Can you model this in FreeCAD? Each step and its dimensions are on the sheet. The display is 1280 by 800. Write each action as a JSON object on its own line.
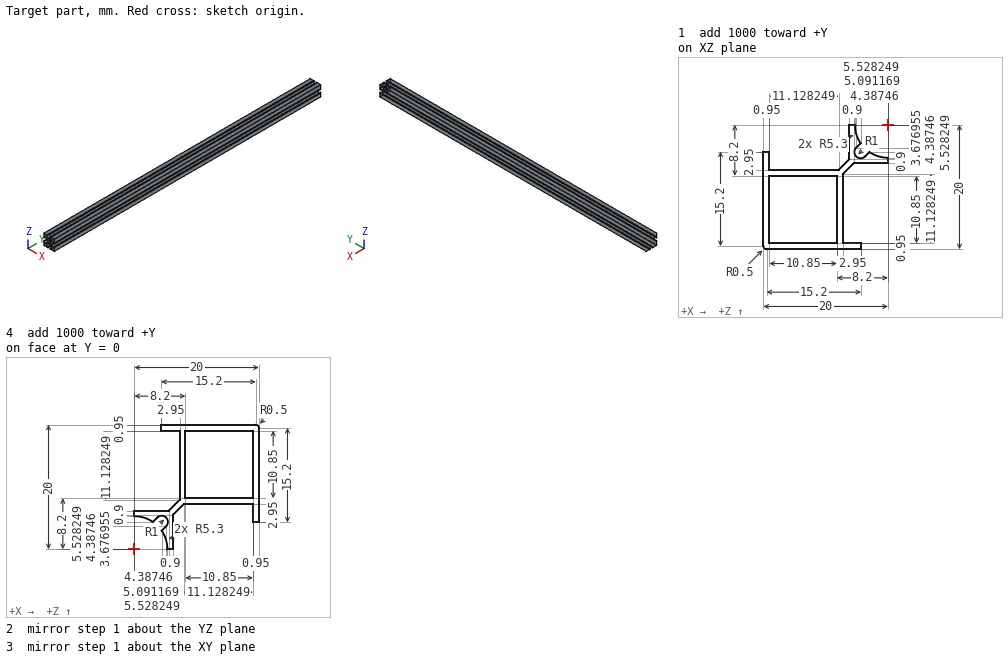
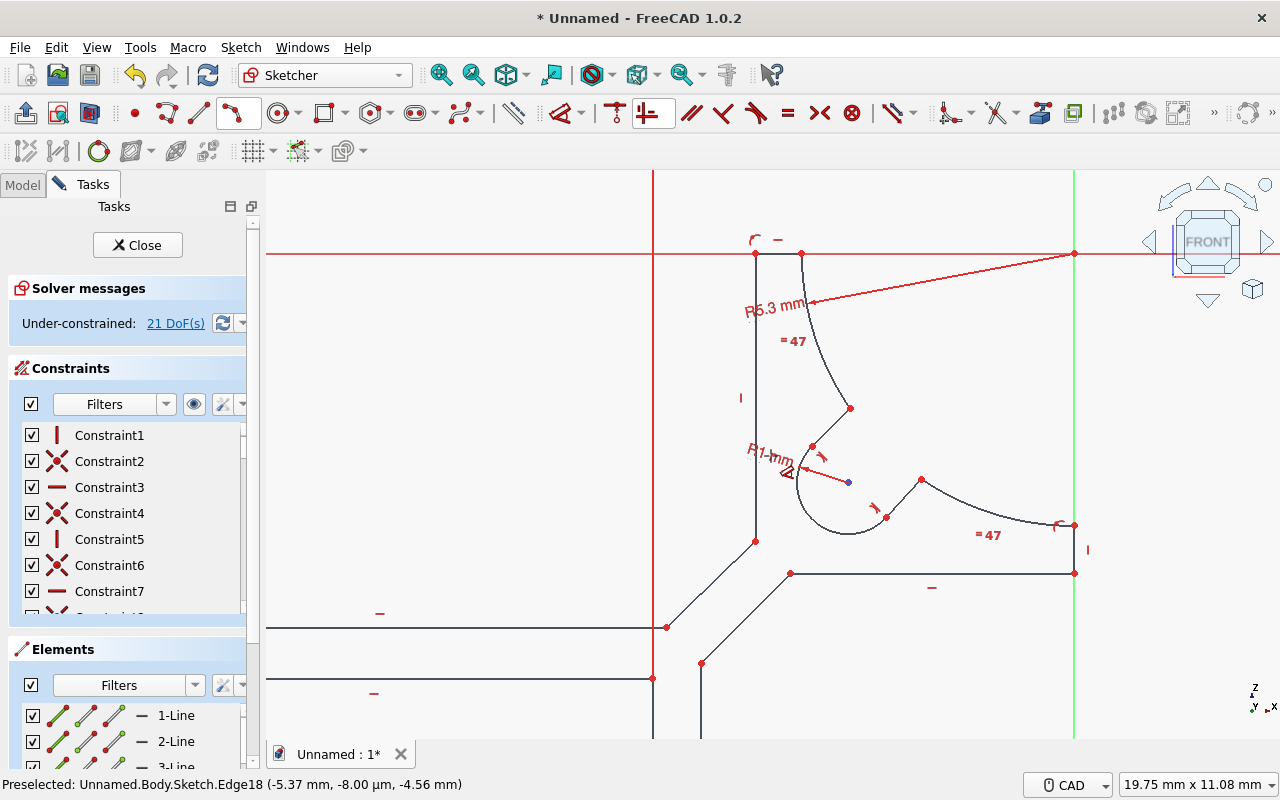
{"action": "scroll", "coordinate": [788, 272], "scroll_direction": "down", "scroll_amount": 5}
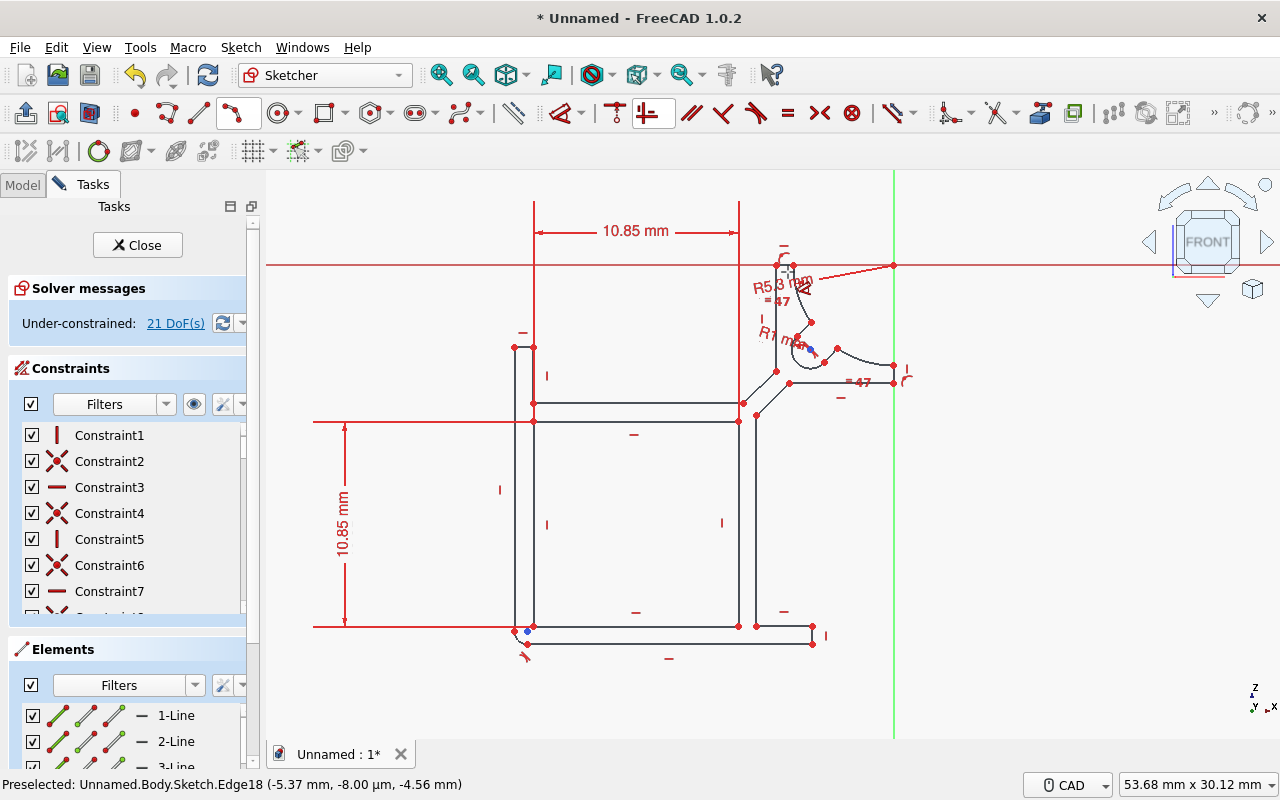
{"action": "scroll", "coordinate": [516, 637], "scroll_direction": "up", "scroll_amount": 8}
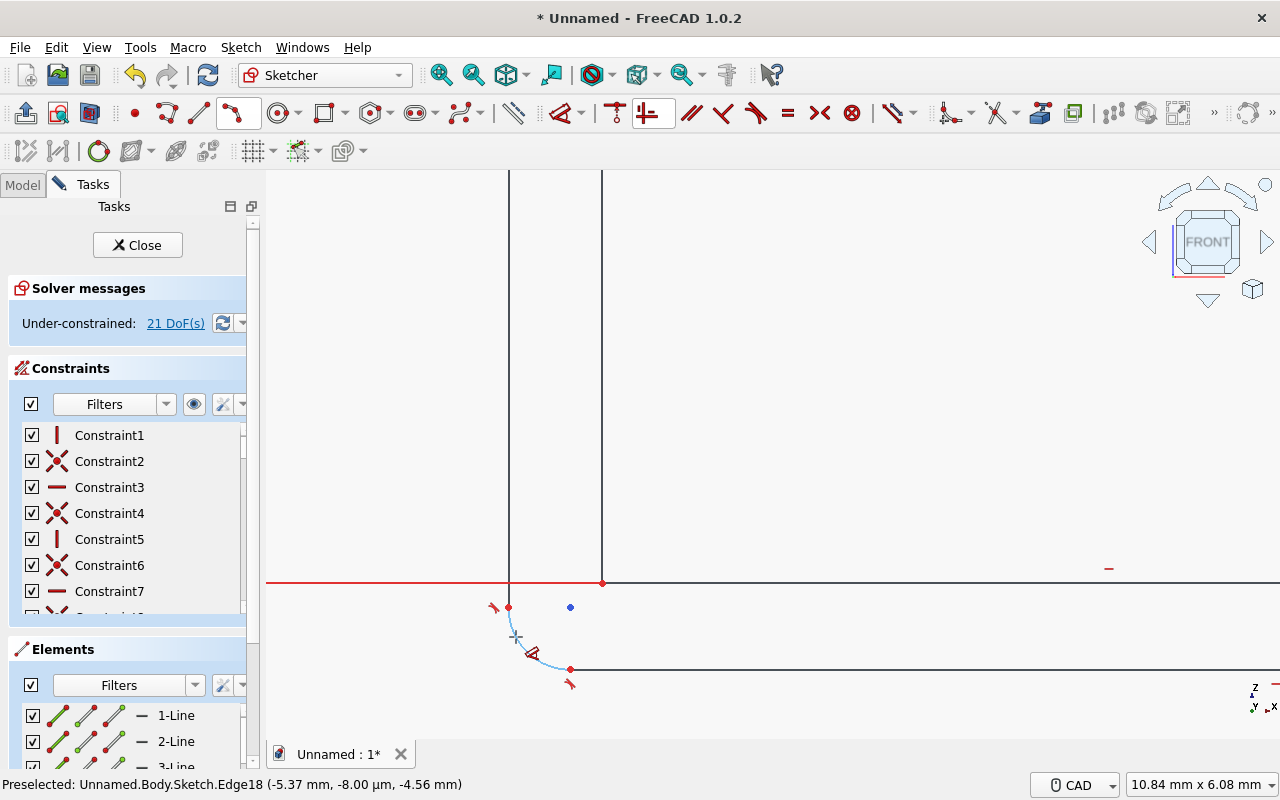
{"action": "left_click", "coordinate": [515, 636]}
{"action": "left_click", "coordinate": [486, 650]}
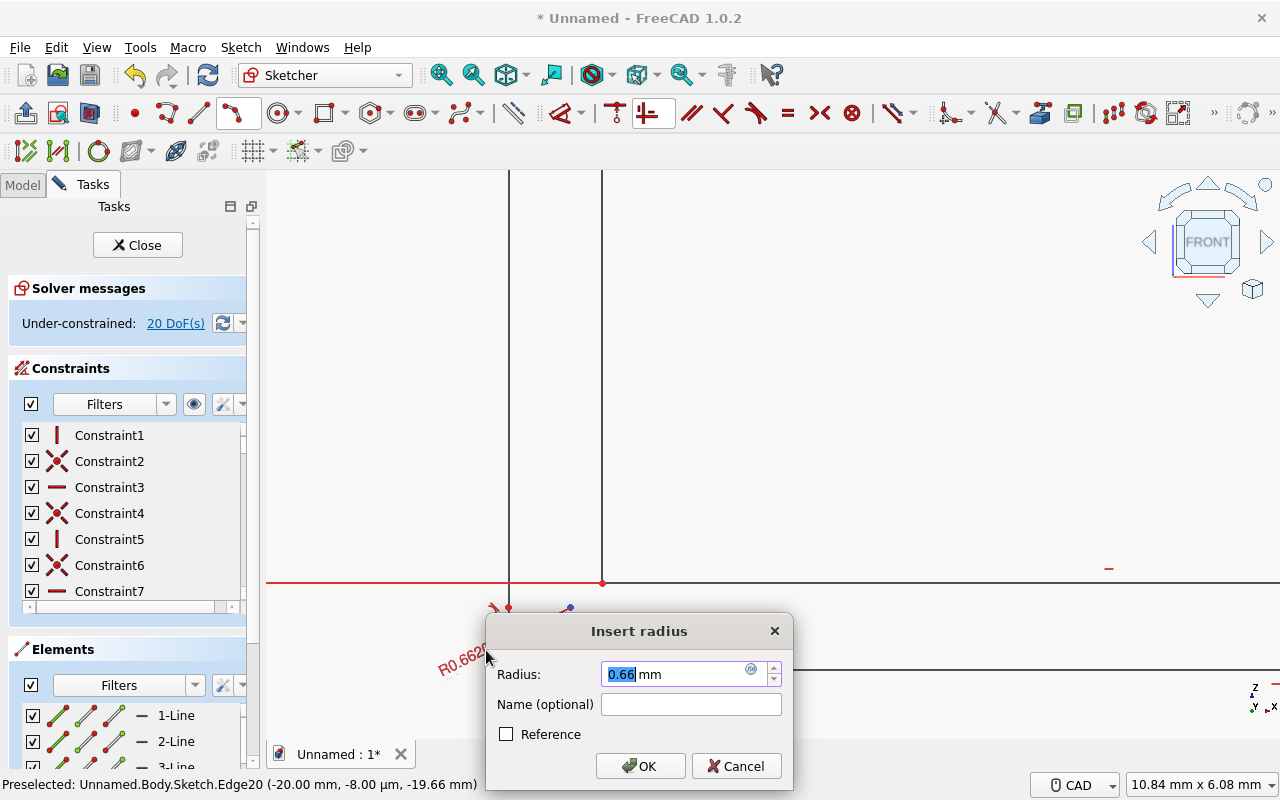
{"action": "type", "text": "0.5"}
{"action": "key", "text": "Return"}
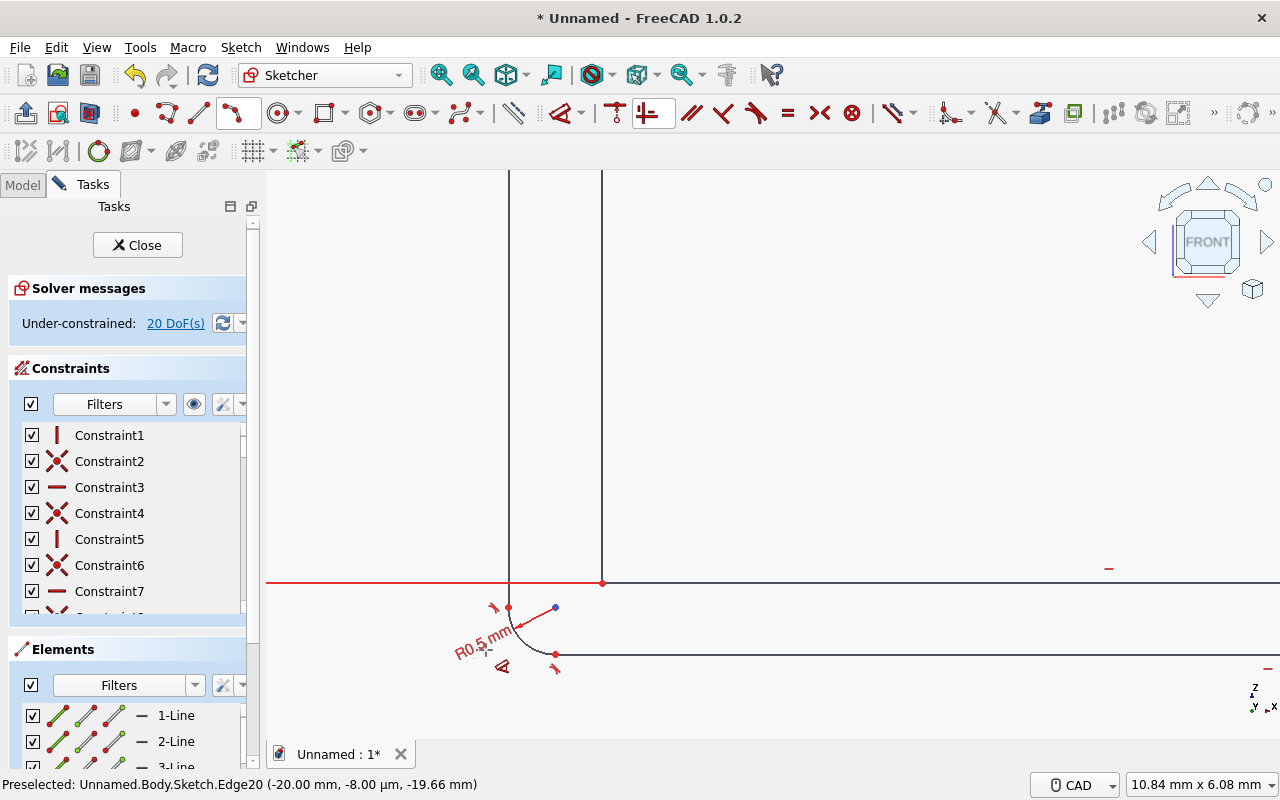
{"action": "scroll", "coordinate": [516, 638], "scroll_direction": "down", "scroll_amount": 8}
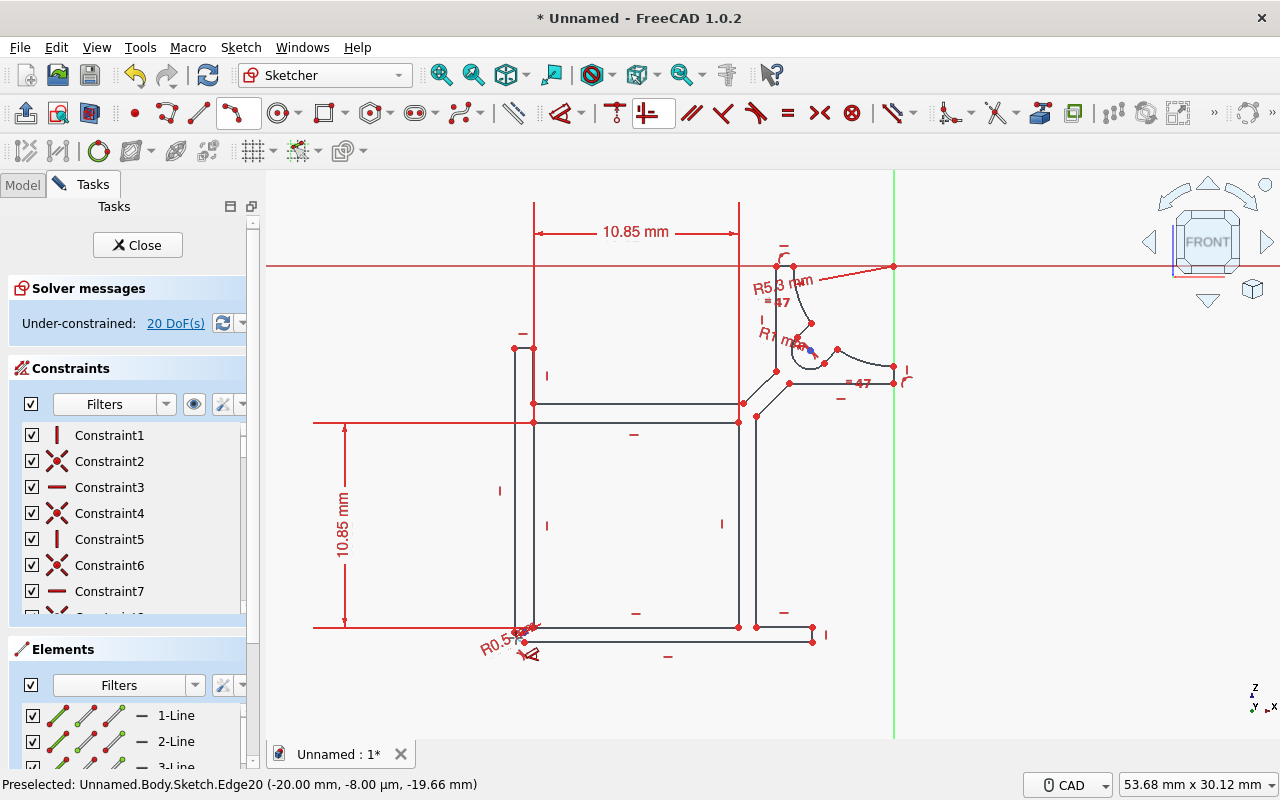
{"action": "scroll", "coordinate": [781, 266], "scroll_direction": "up", "scroll_amount": 5}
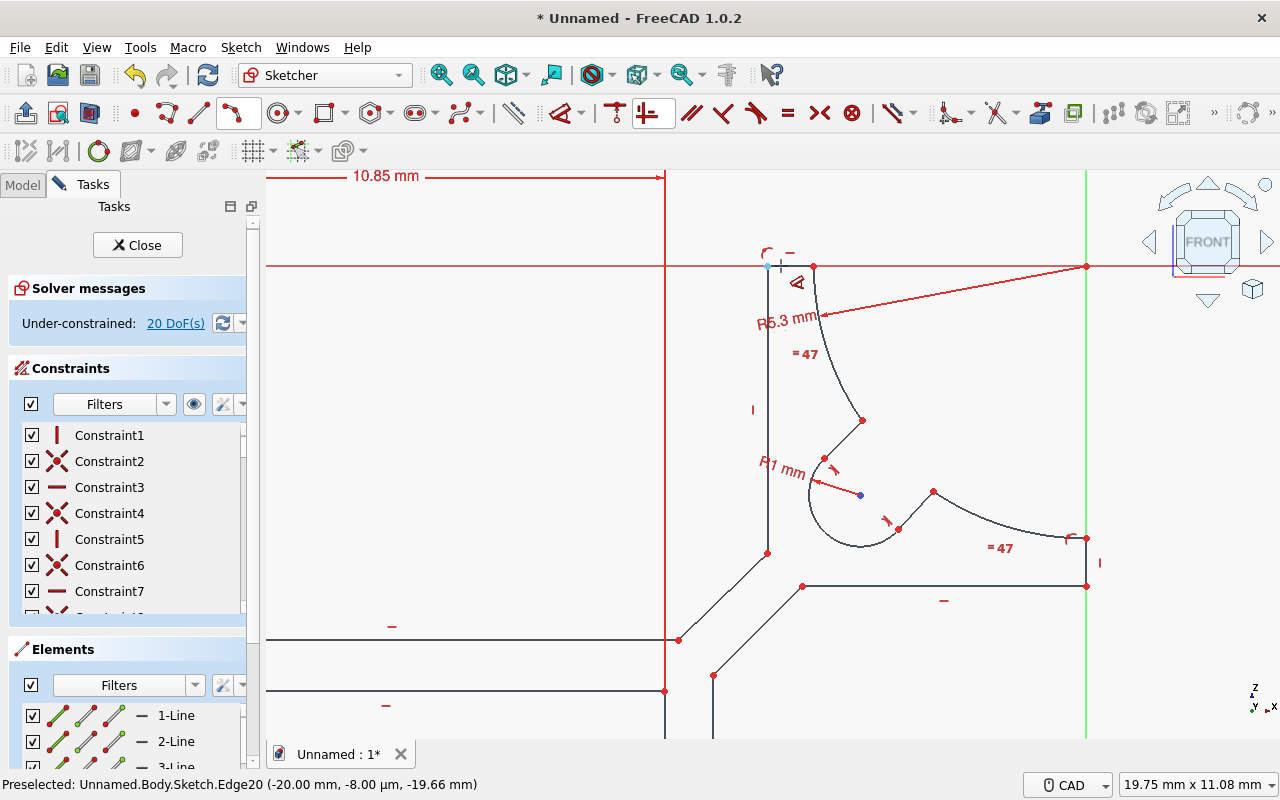
{"action": "left_click", "coordinate": [781, 266]}
{"action": "left_click", "coordinate": [791, 232]}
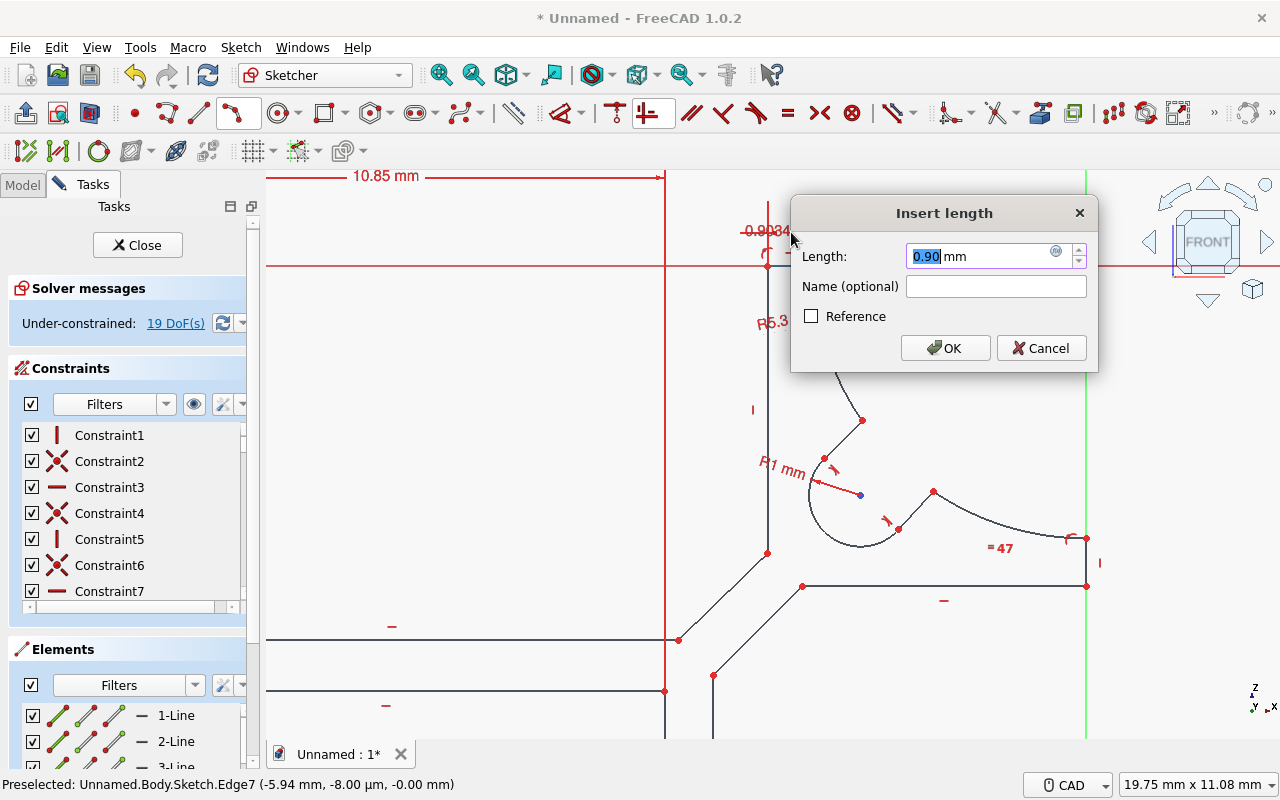
{"action": "type", "text": "0.9"}
{"action": "key", "text": "Return"}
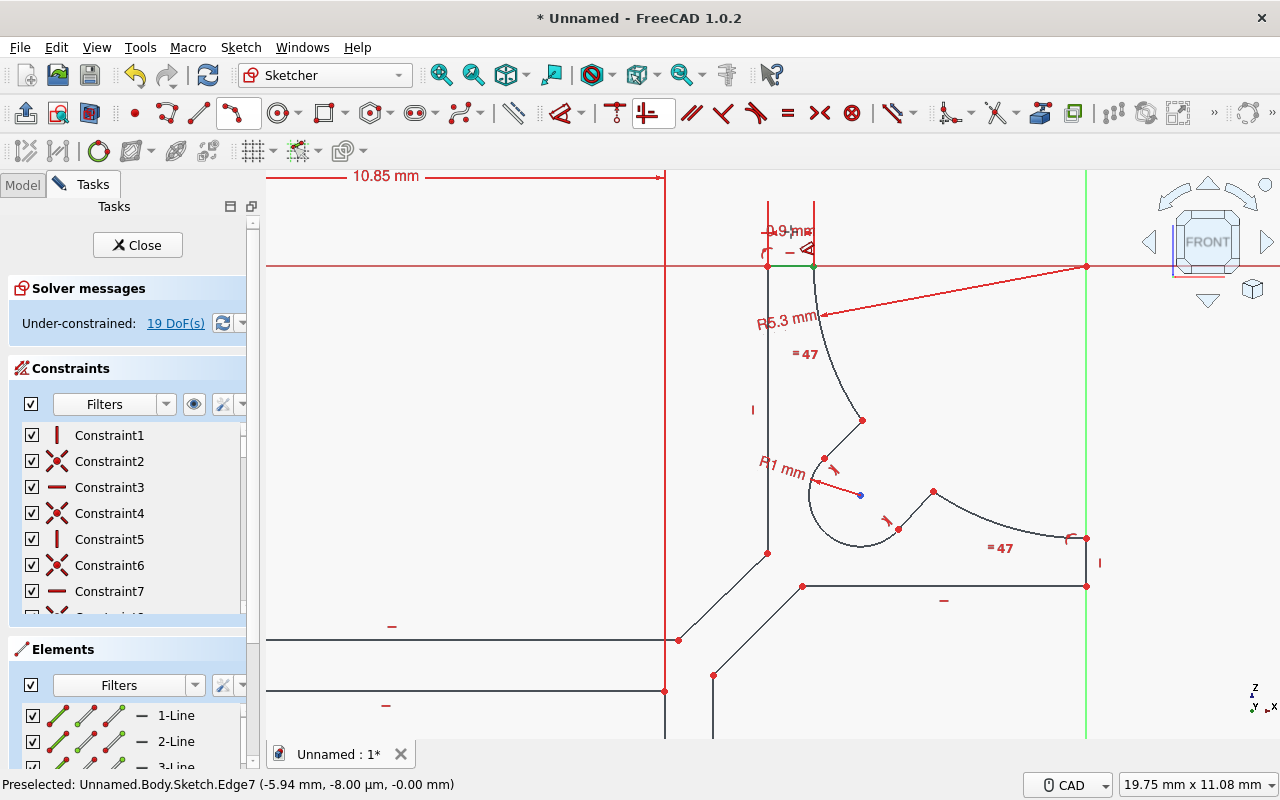
{"action": "left_click", "coordinate": [1086, 553]}
{"action": "left_click", "coordinate": [1052, 562]}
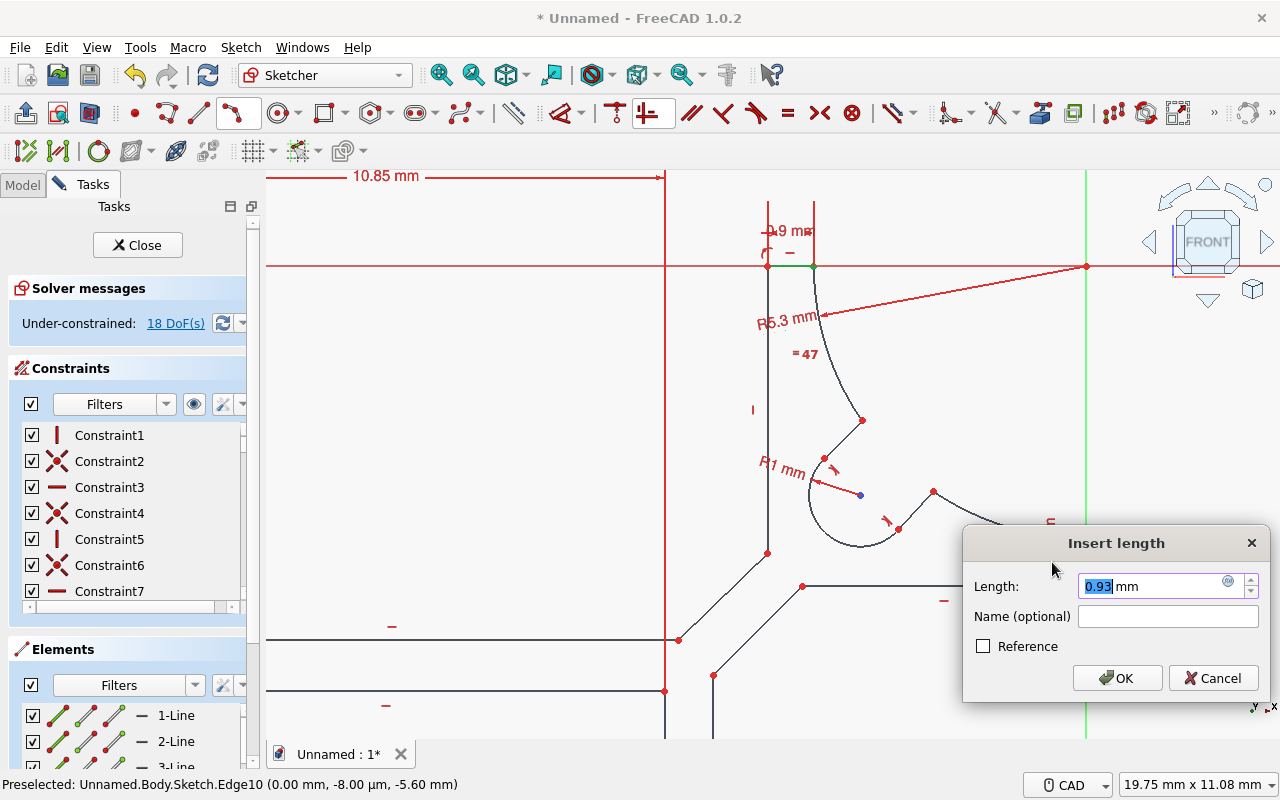
{"action": "type", "text": "0.9"}
{"action": "key", "text": "Return"}